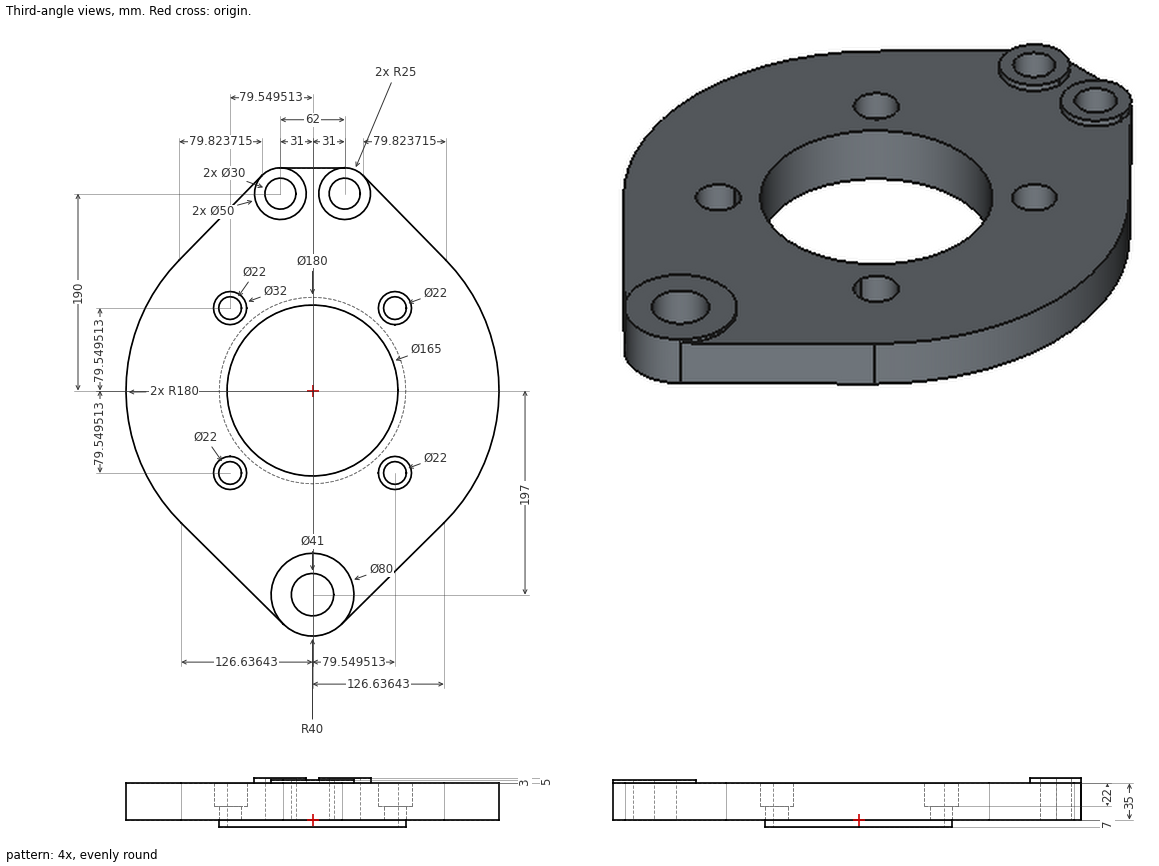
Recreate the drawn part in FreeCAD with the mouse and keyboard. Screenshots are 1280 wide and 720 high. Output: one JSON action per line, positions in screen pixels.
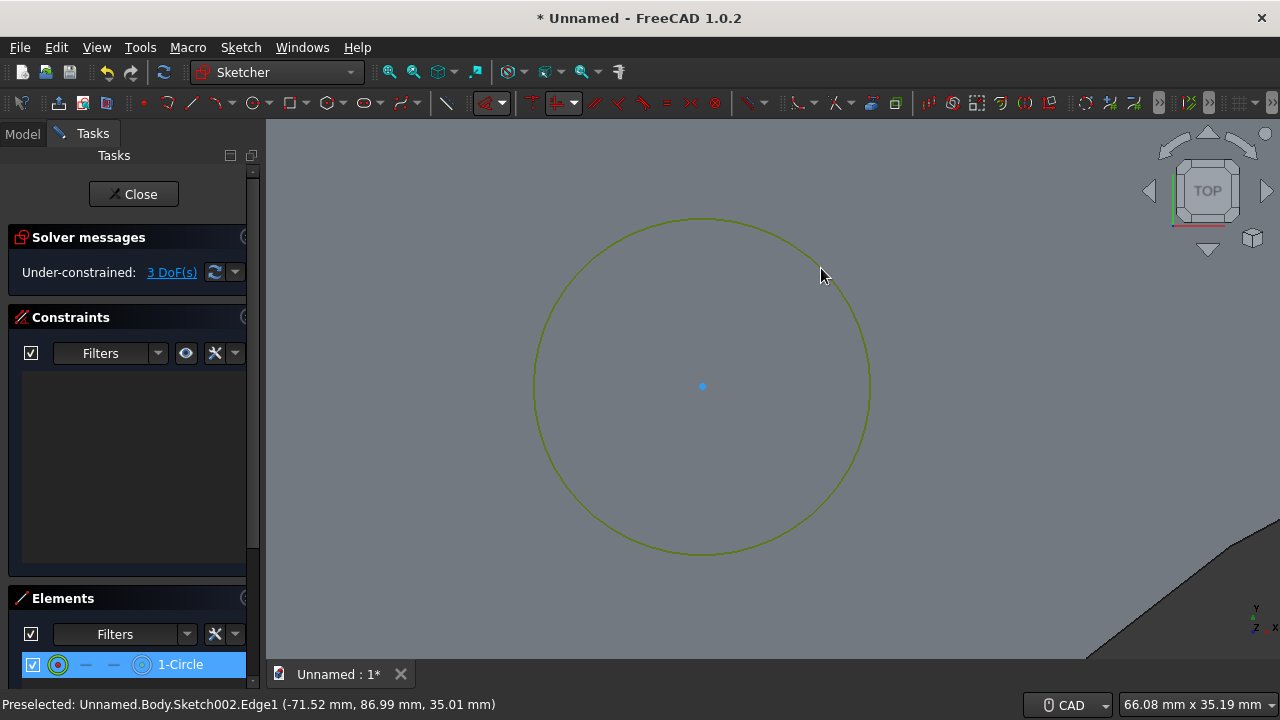
{"action": "key", "text": "k o"}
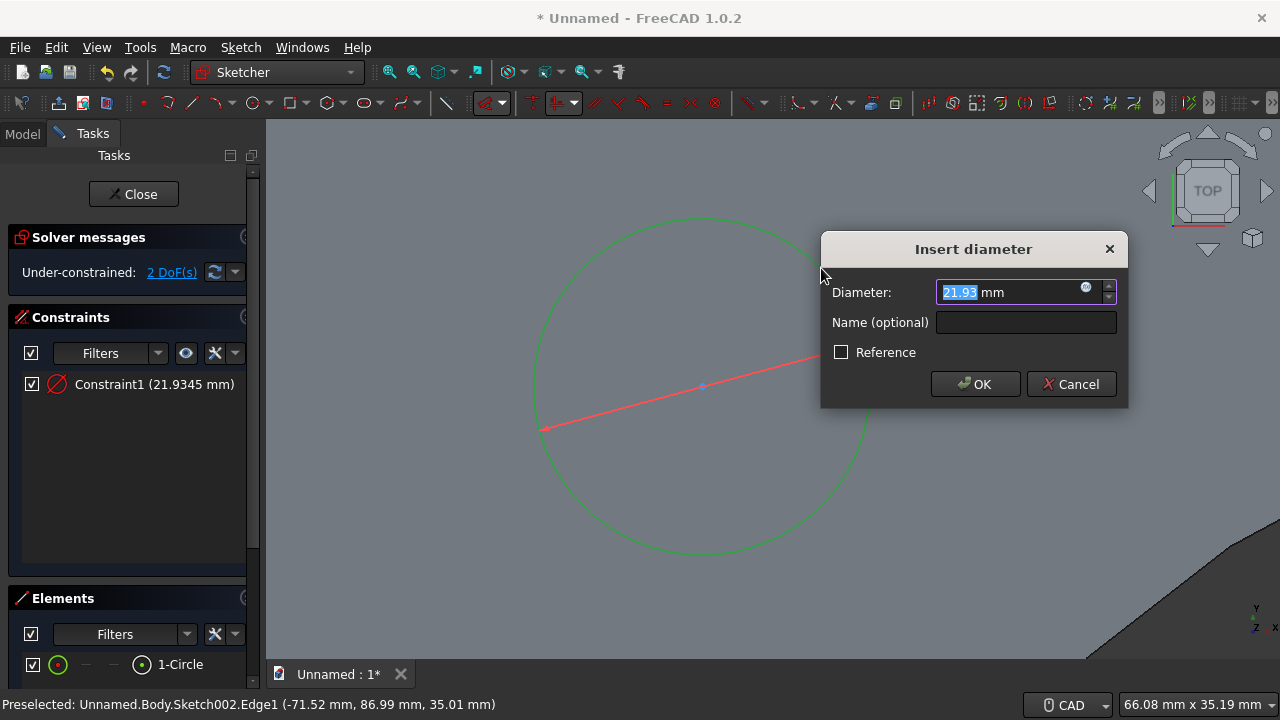
{"action": "type", "text": "22"}
{"action": "key", "text": "Return"}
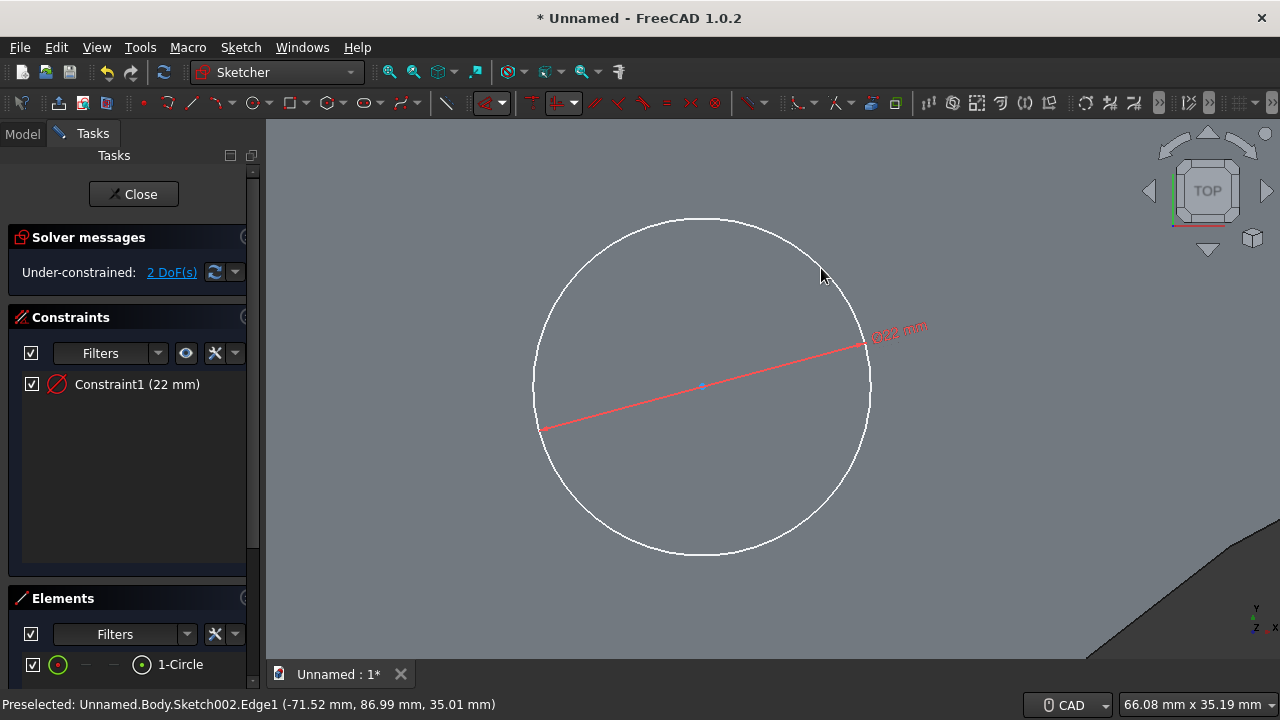
{"action": "left_click", "coordinate": [702, 387]}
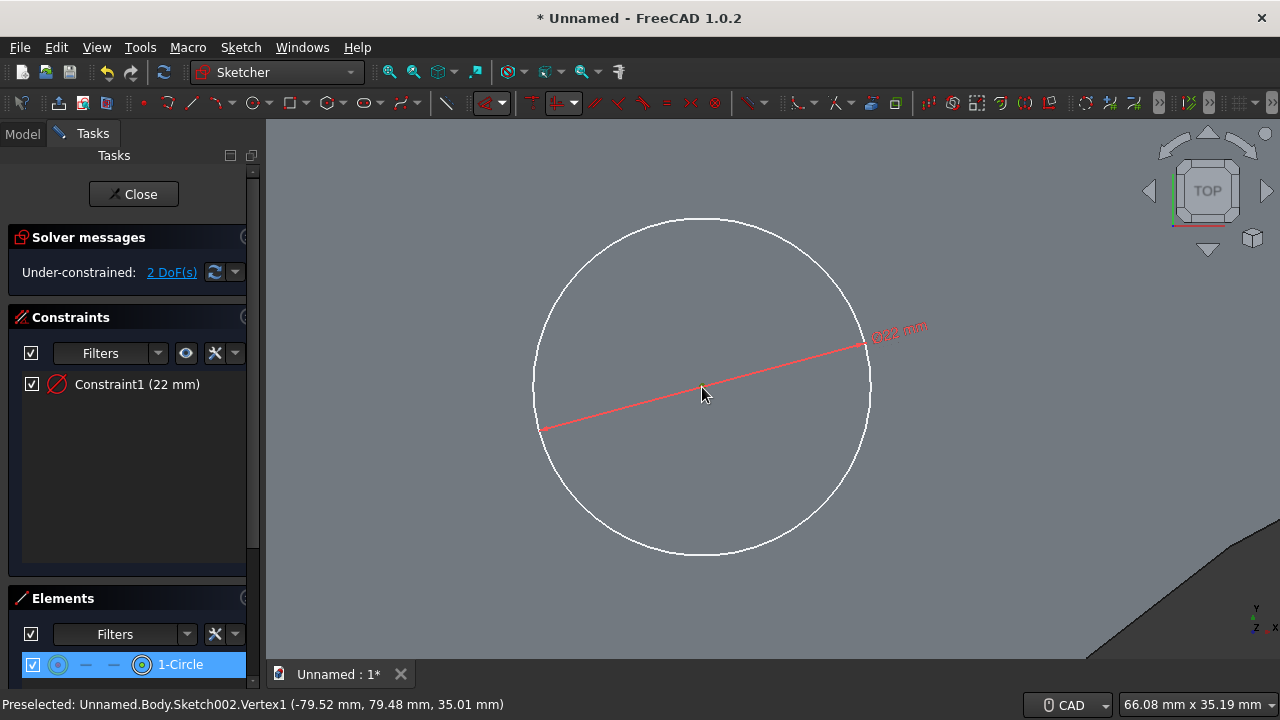
{"action": "key", "text": "l"}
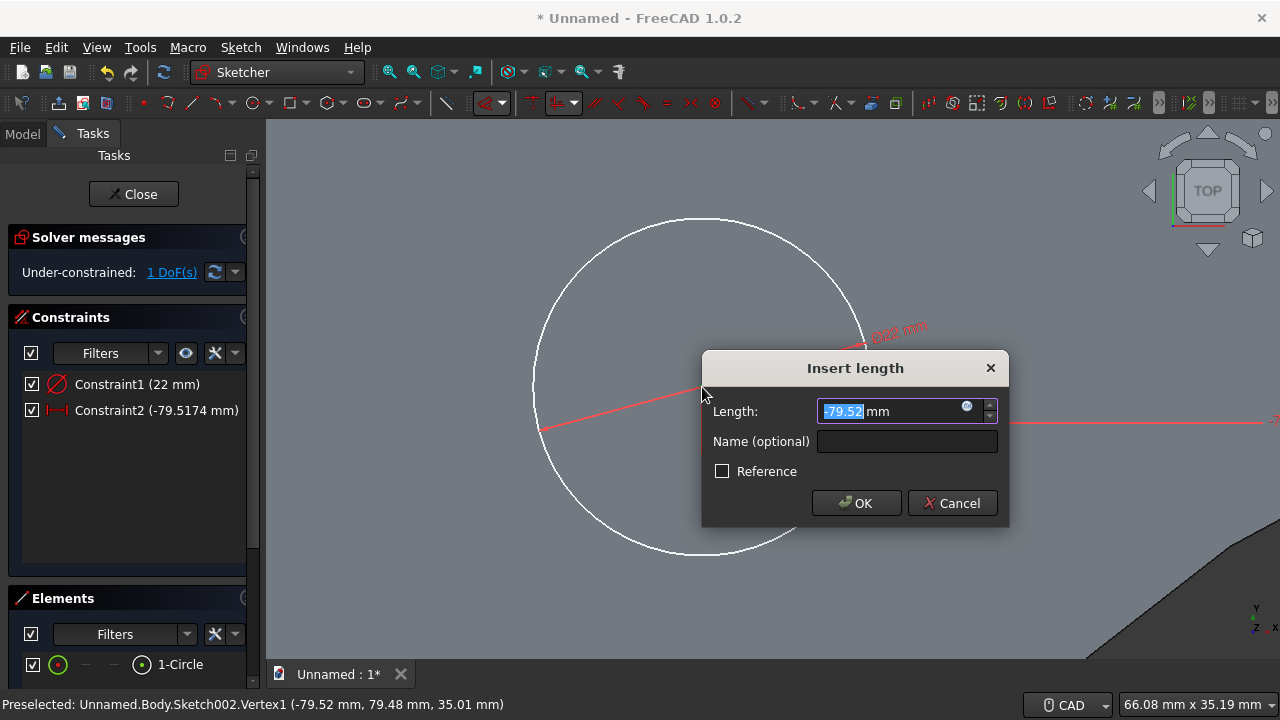
{"action": "type", "text": "-79.549513"}
{"action": "key", "text": "Return"}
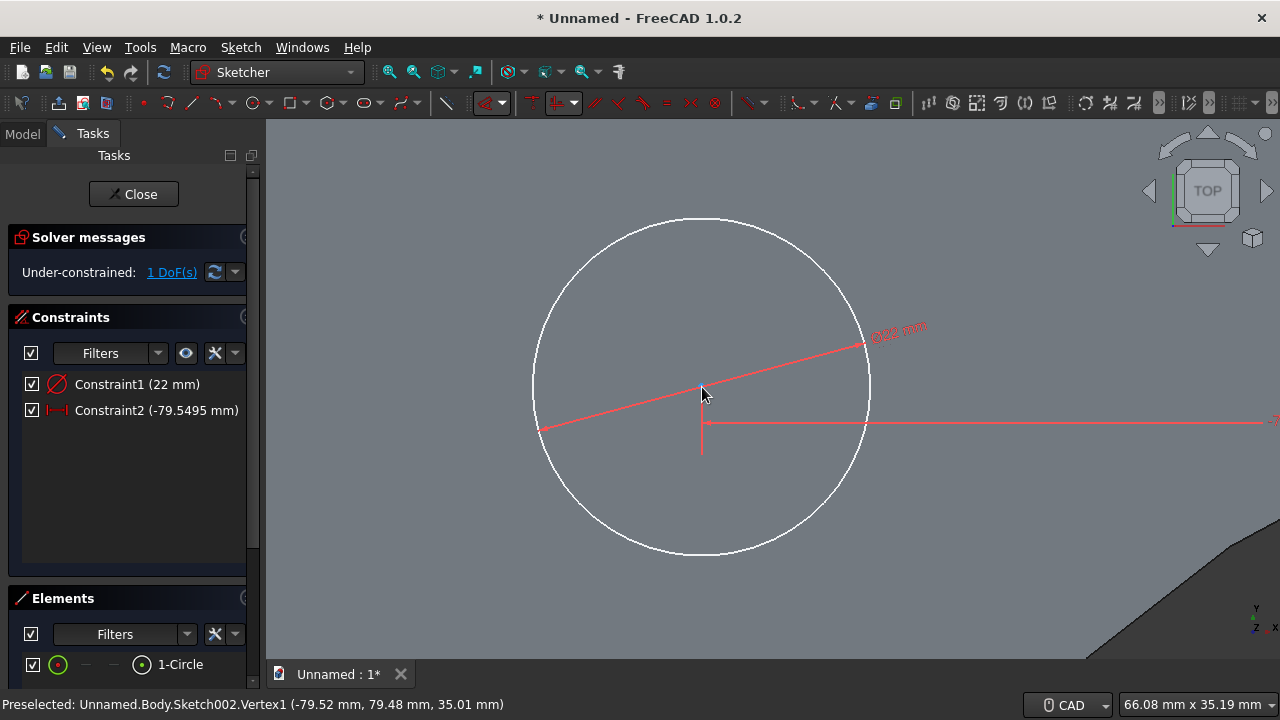
{"action": "left_click", "coordinate": [702, 387]}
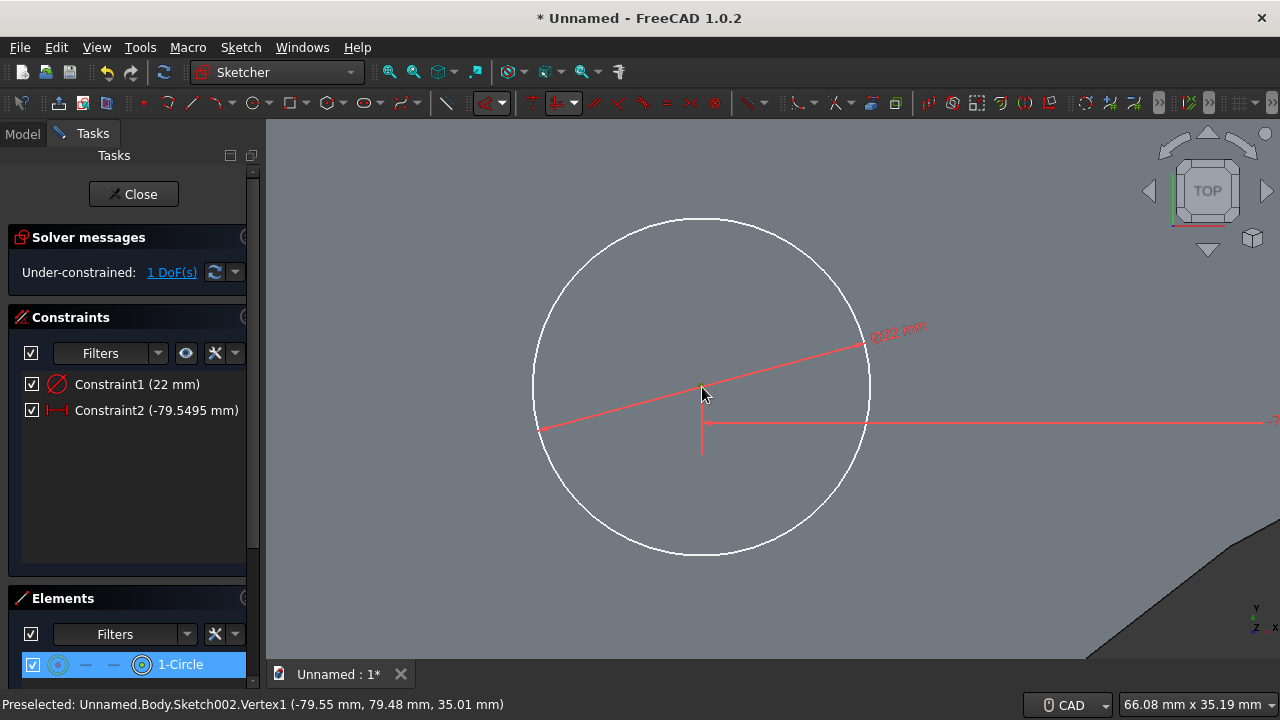
{"action": "left_click", "coordinate": [504, 104]}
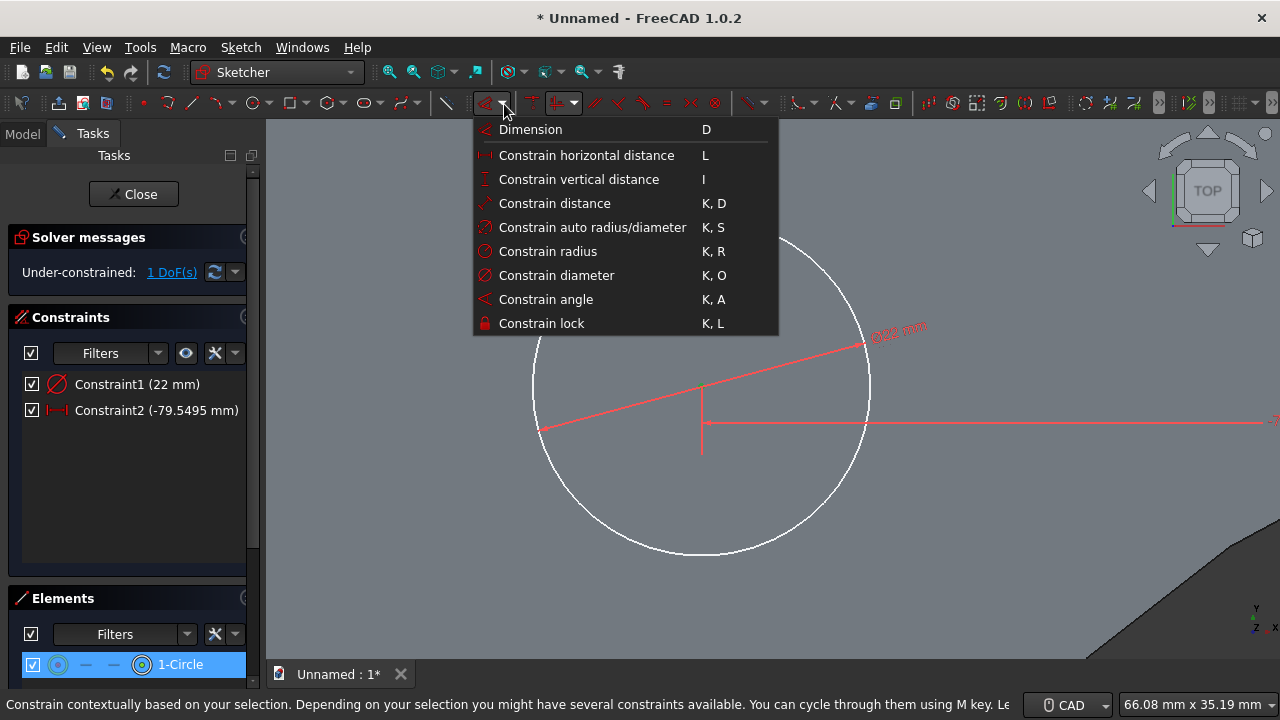
{"action": "left_click", "coordinate": [626, 179]}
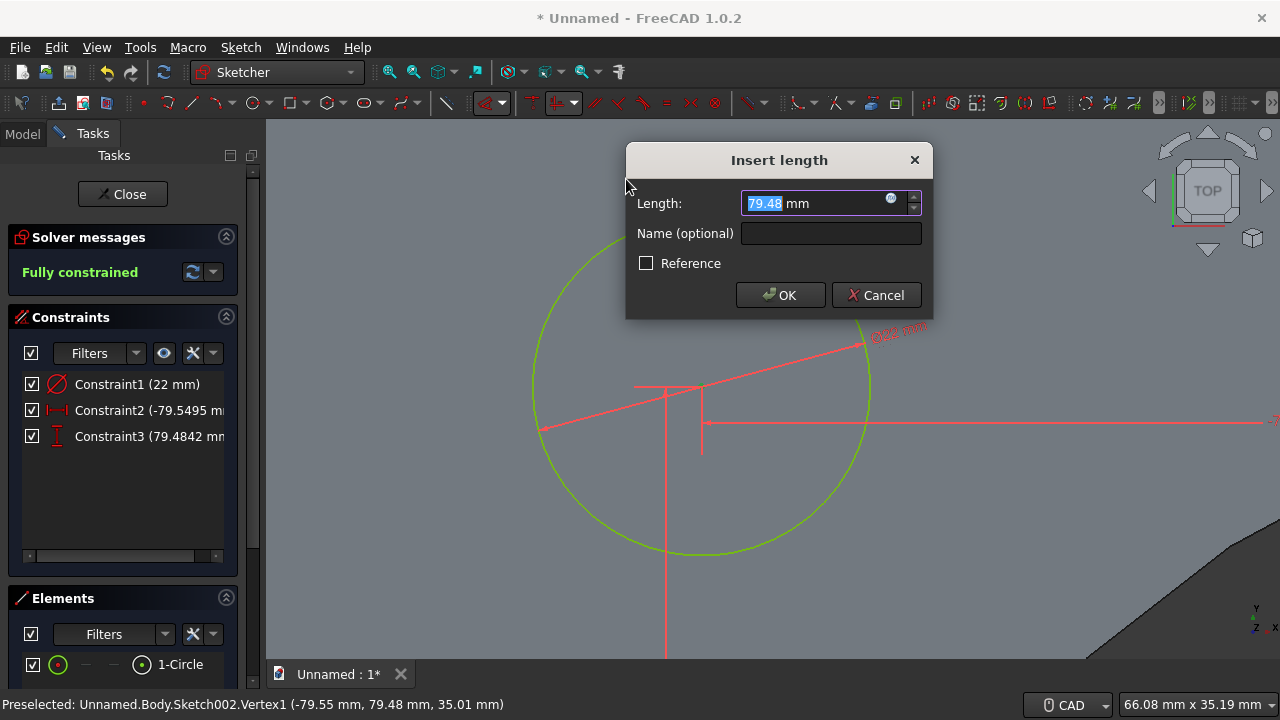
{"action": "type", "text": "79.549513"}
{"action": "key", "text": "Return"}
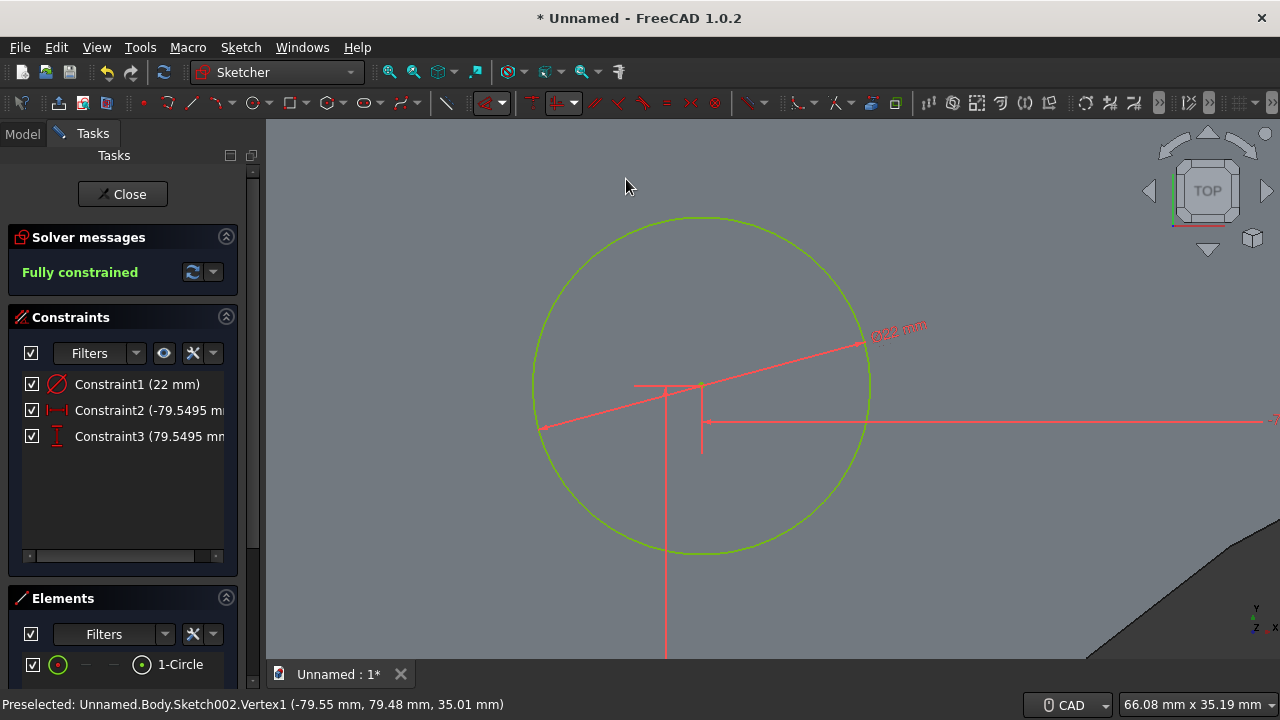
{"action": "left_click", "coordinate": [123, 194]}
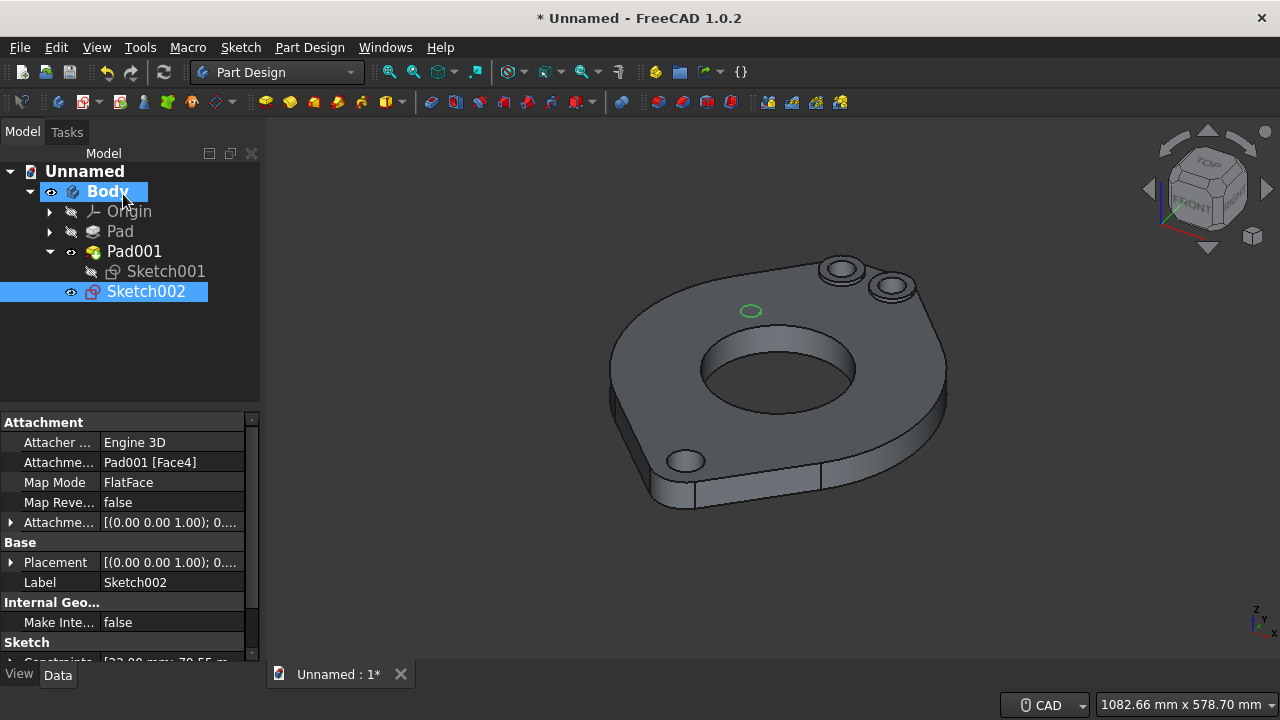
{"action": "left_click", "coordinate": [432, 102]}